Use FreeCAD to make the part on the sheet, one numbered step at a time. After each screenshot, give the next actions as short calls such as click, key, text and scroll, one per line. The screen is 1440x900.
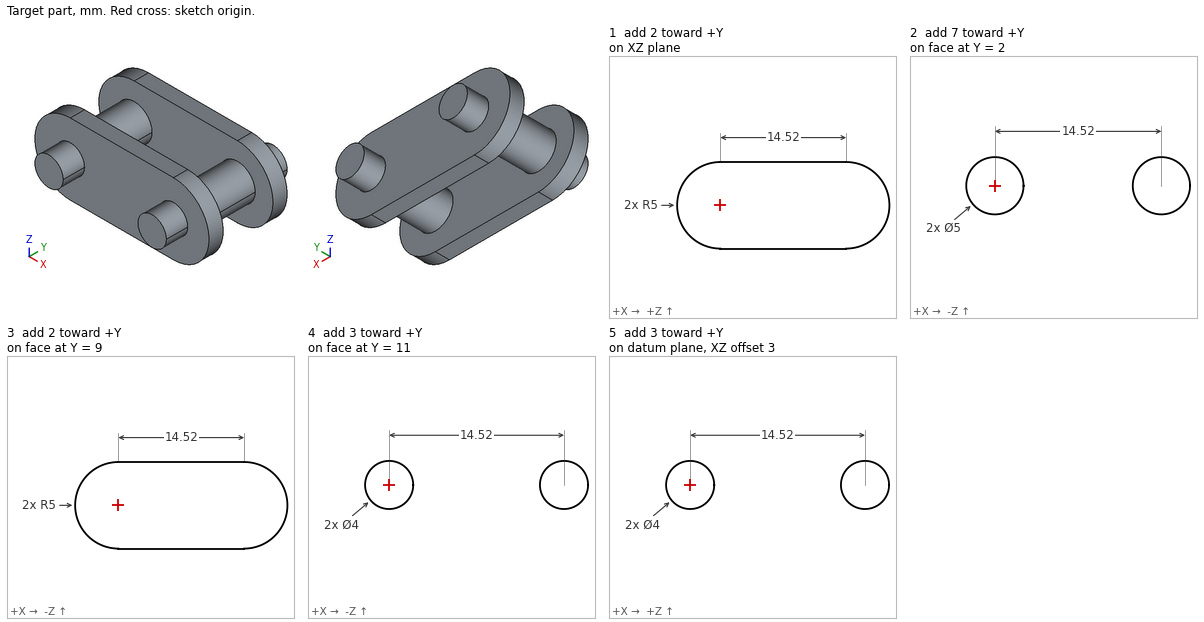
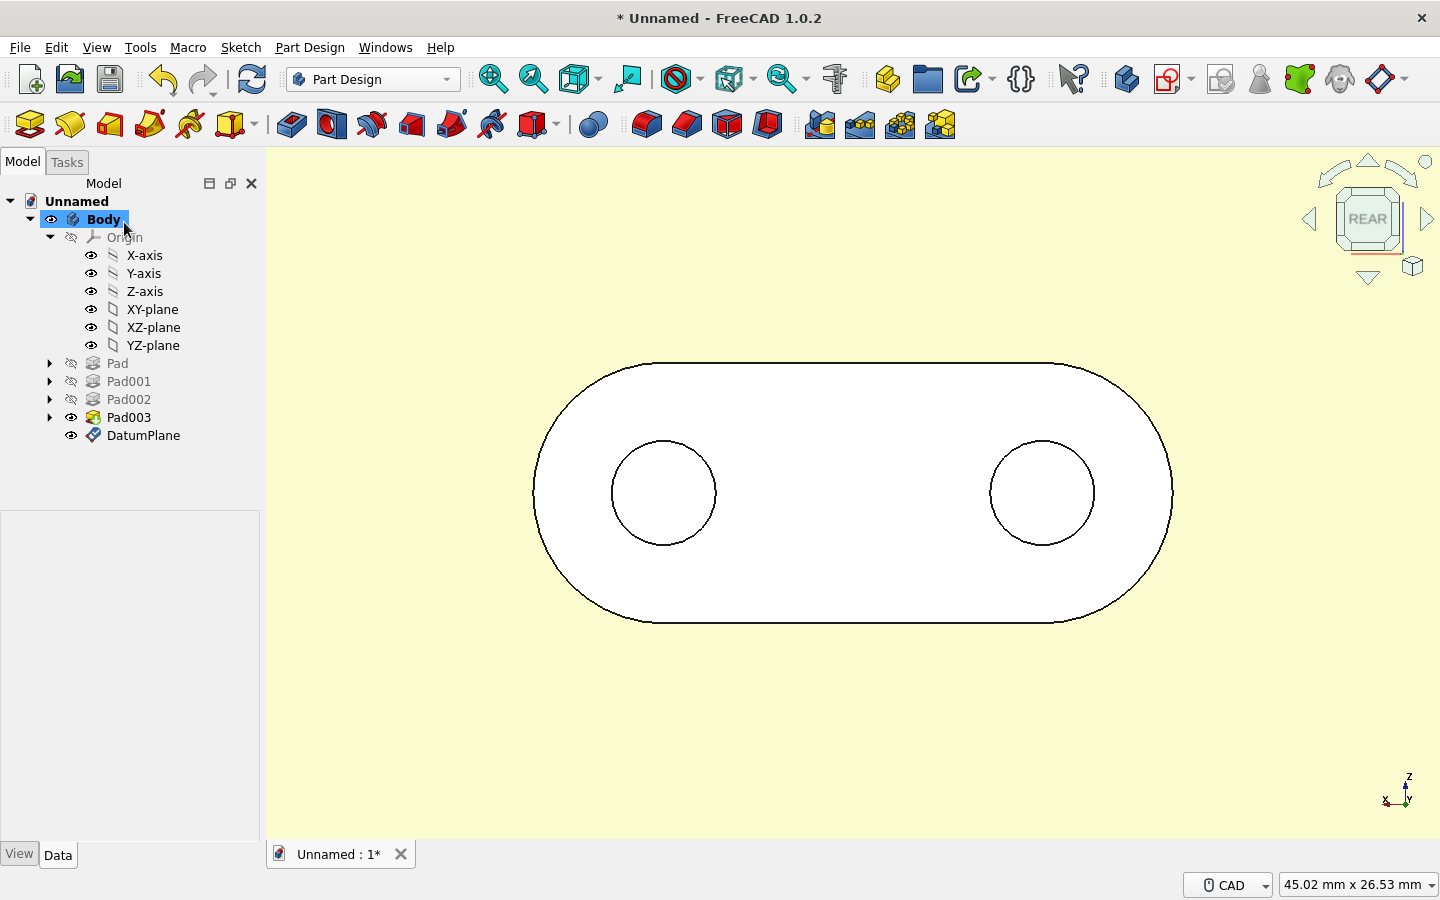
click(116, 435)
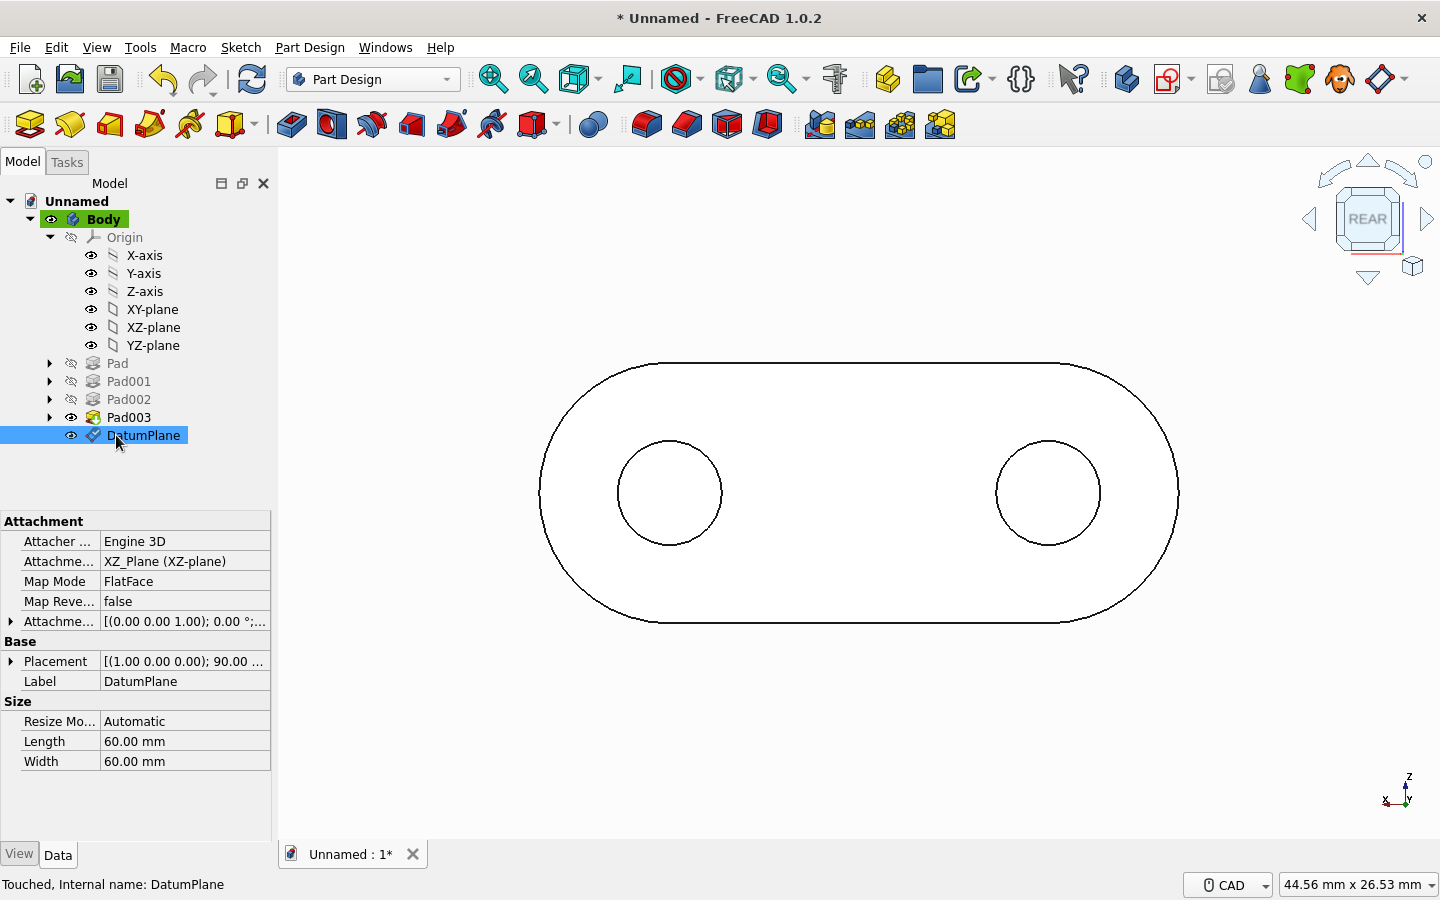
click(1168, 80)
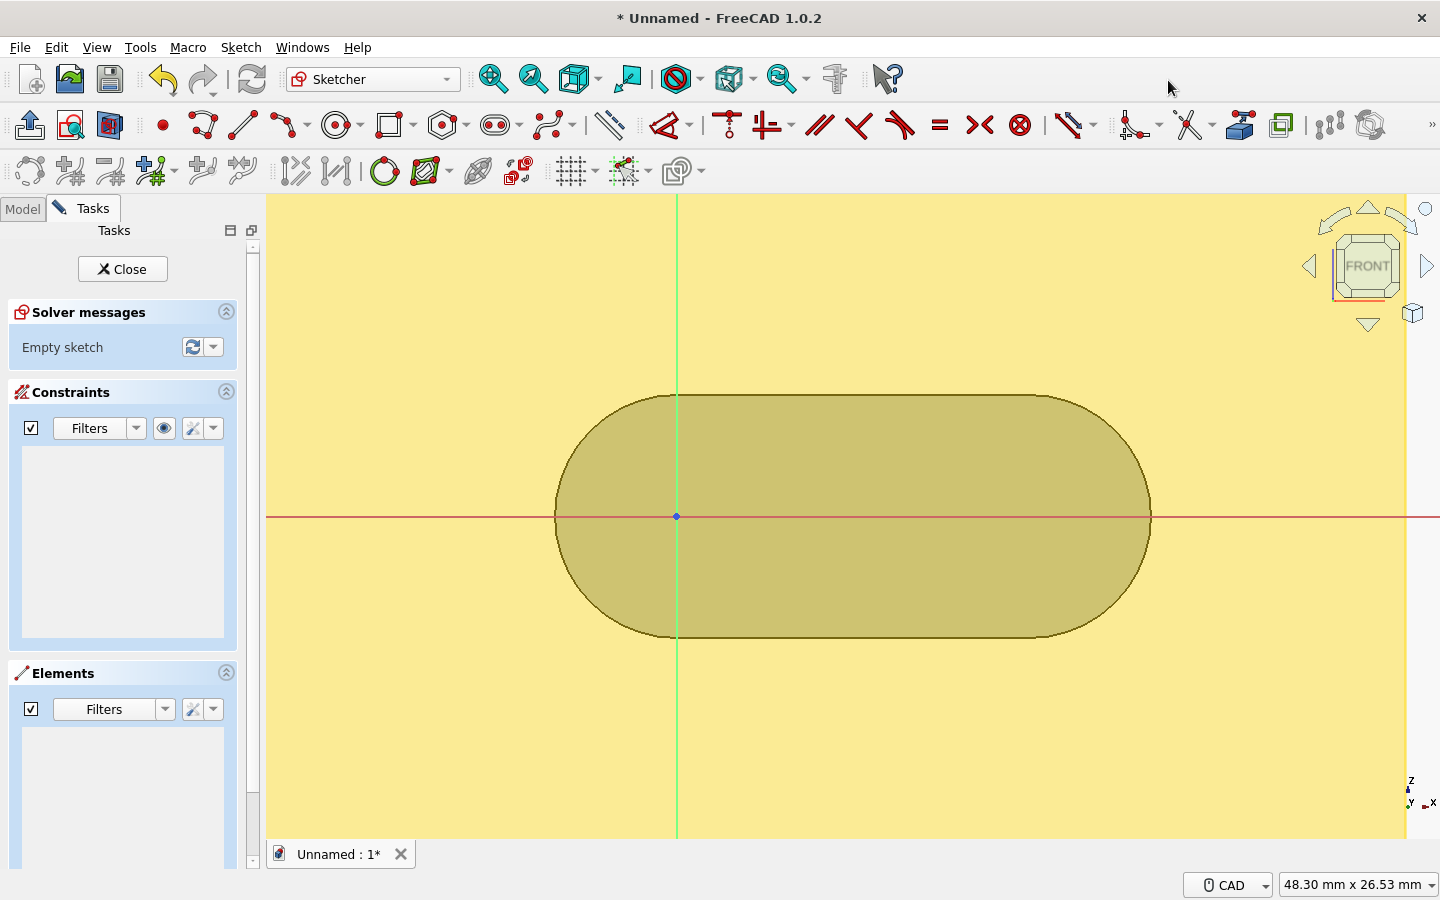
scroll(992, 517, up, 2)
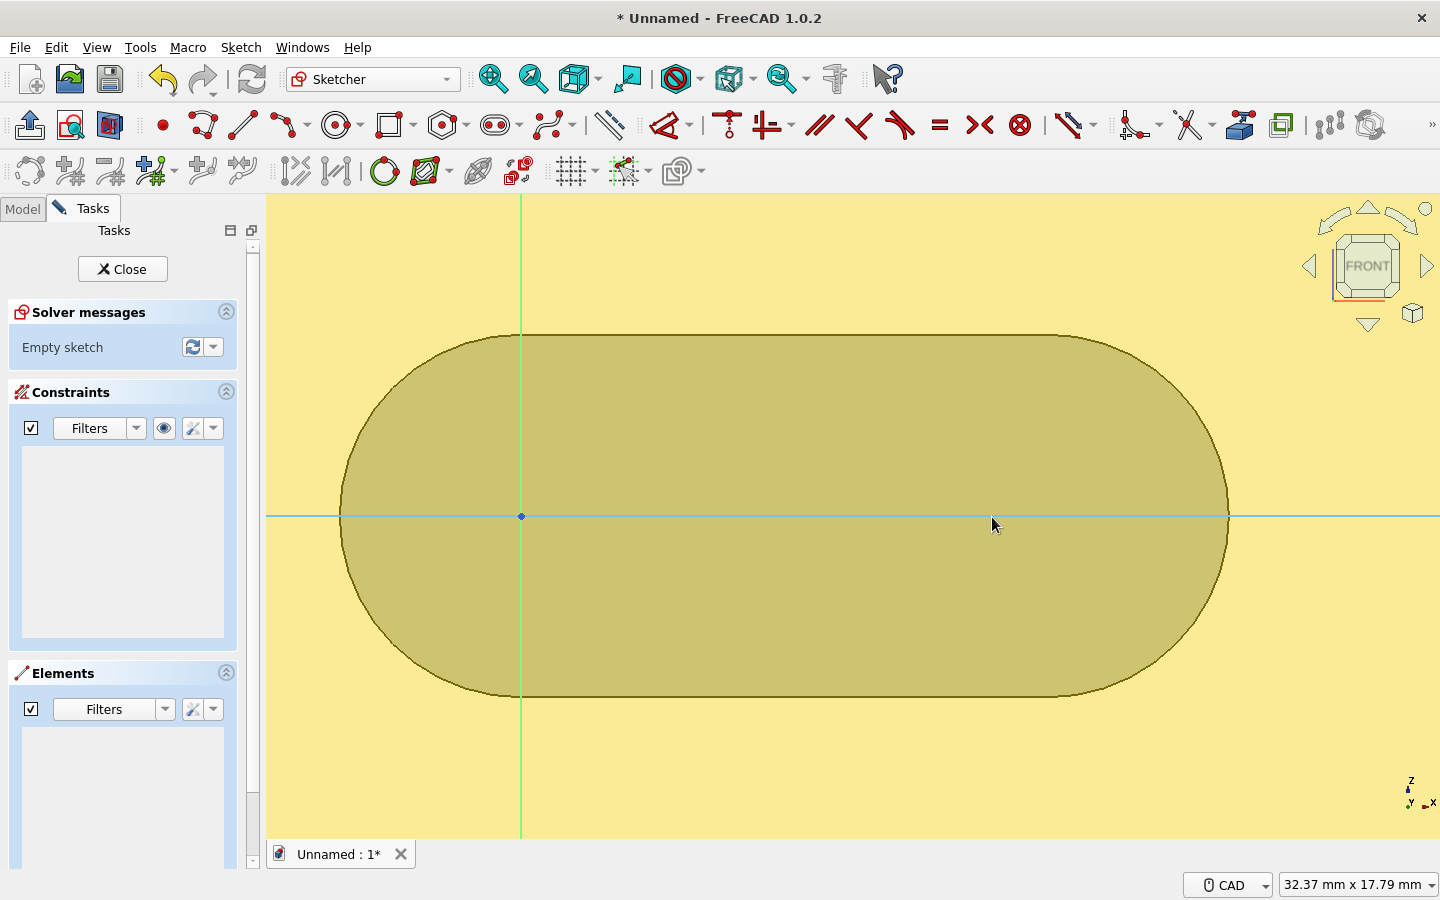
key(g)
key(c)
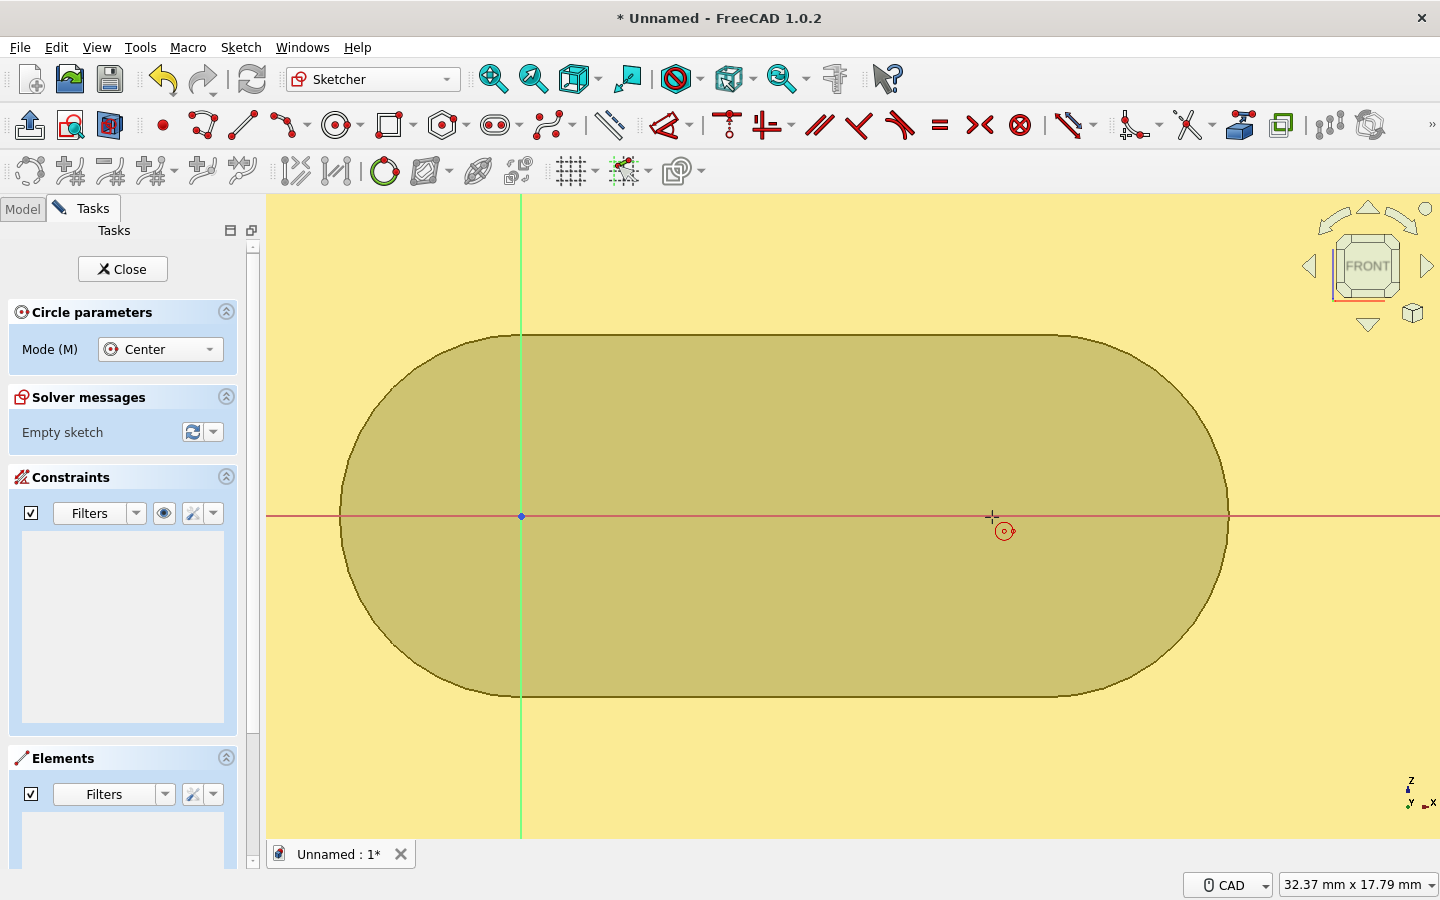
click(521, 516)
move(572, 465)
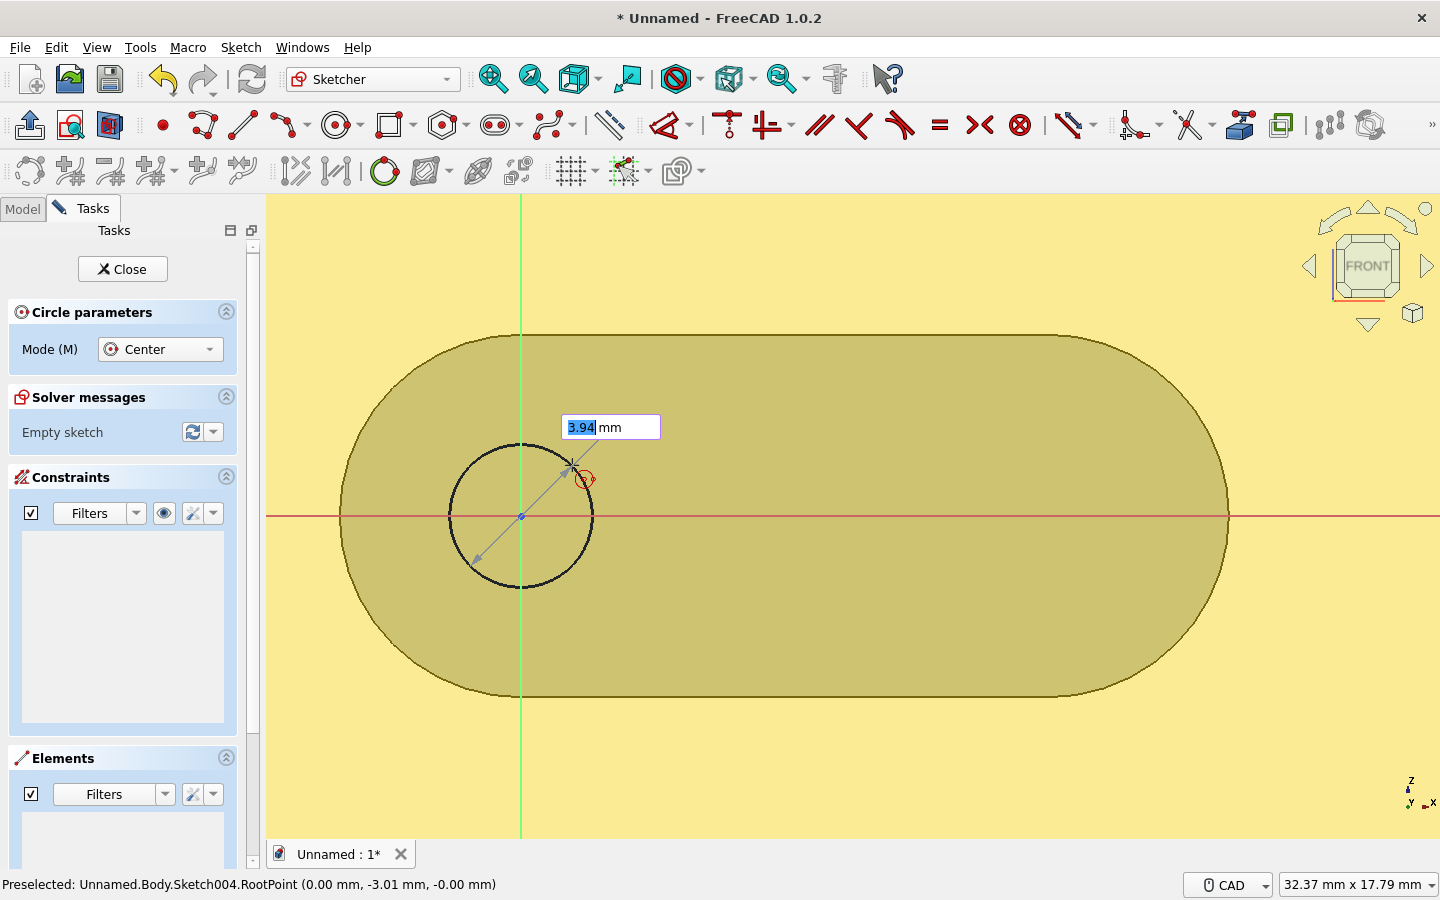
text(4)
key(Return)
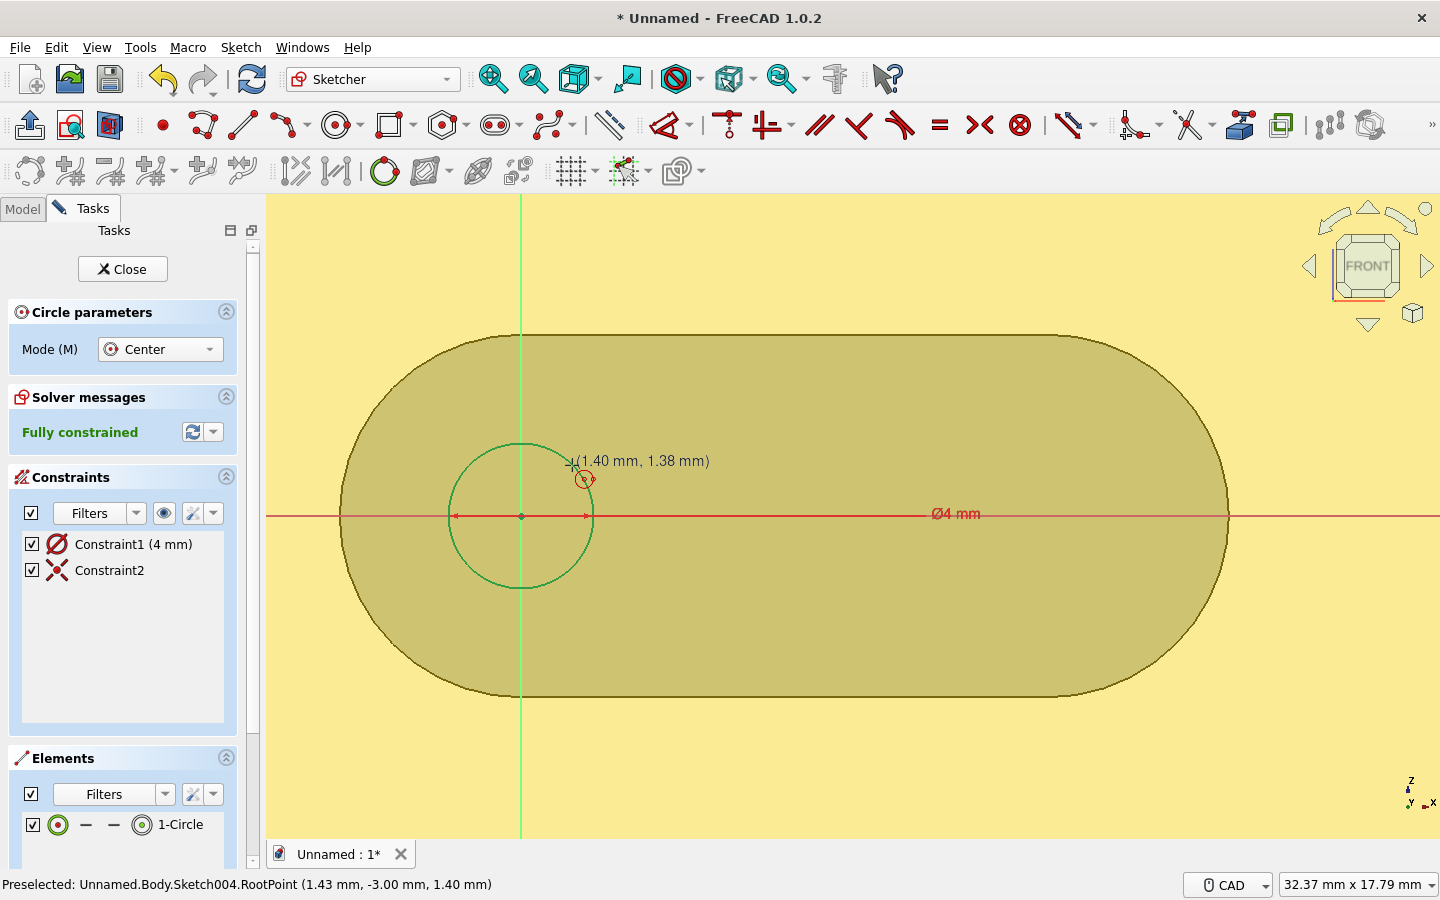
click(1048, 516)
move(1099, 465)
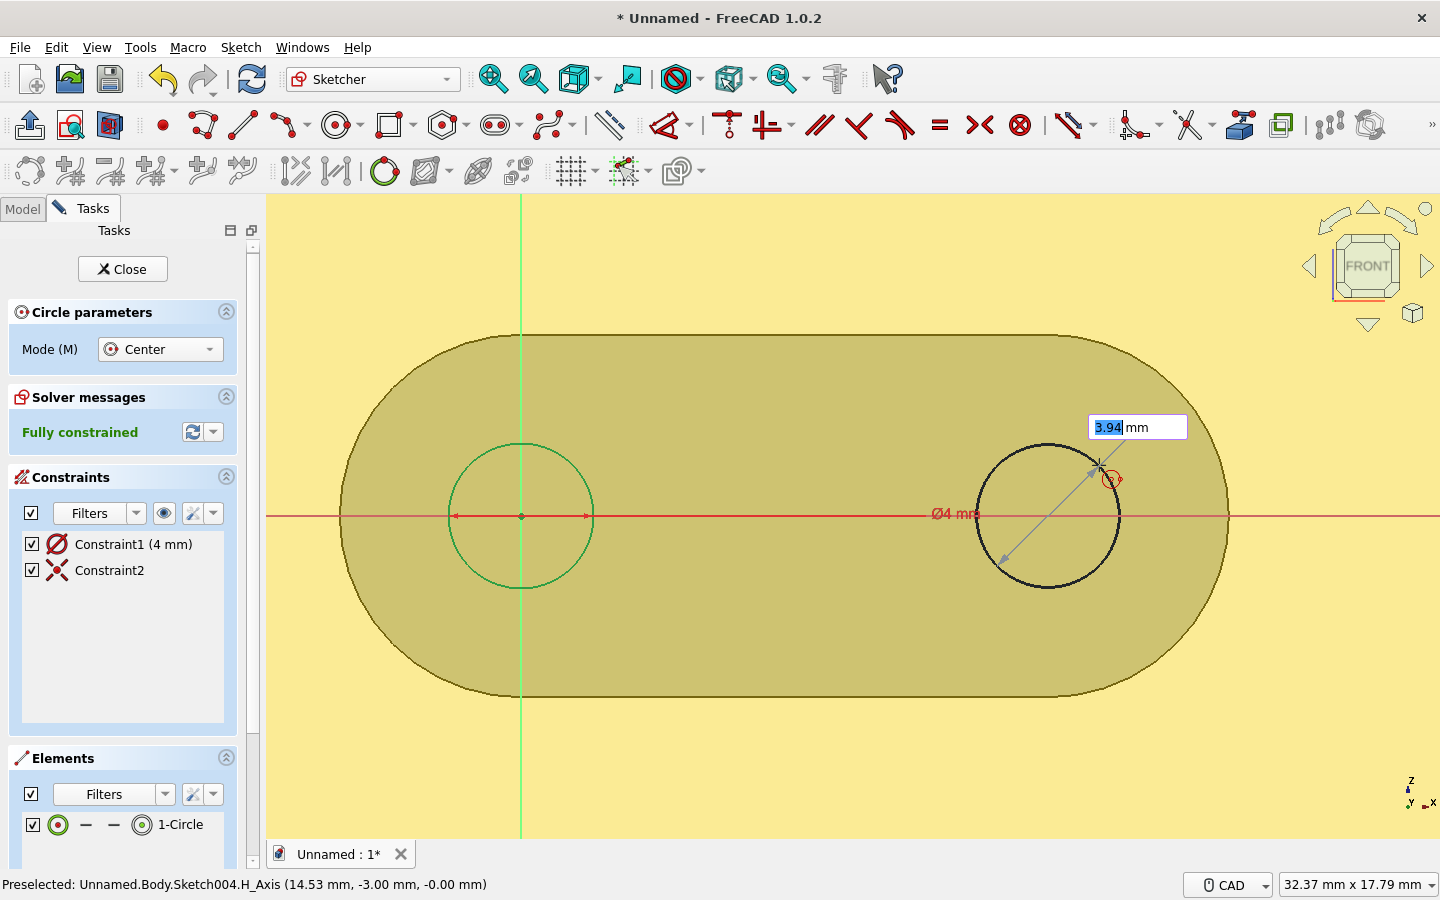
text(4)
key(Return)
key(Escape)